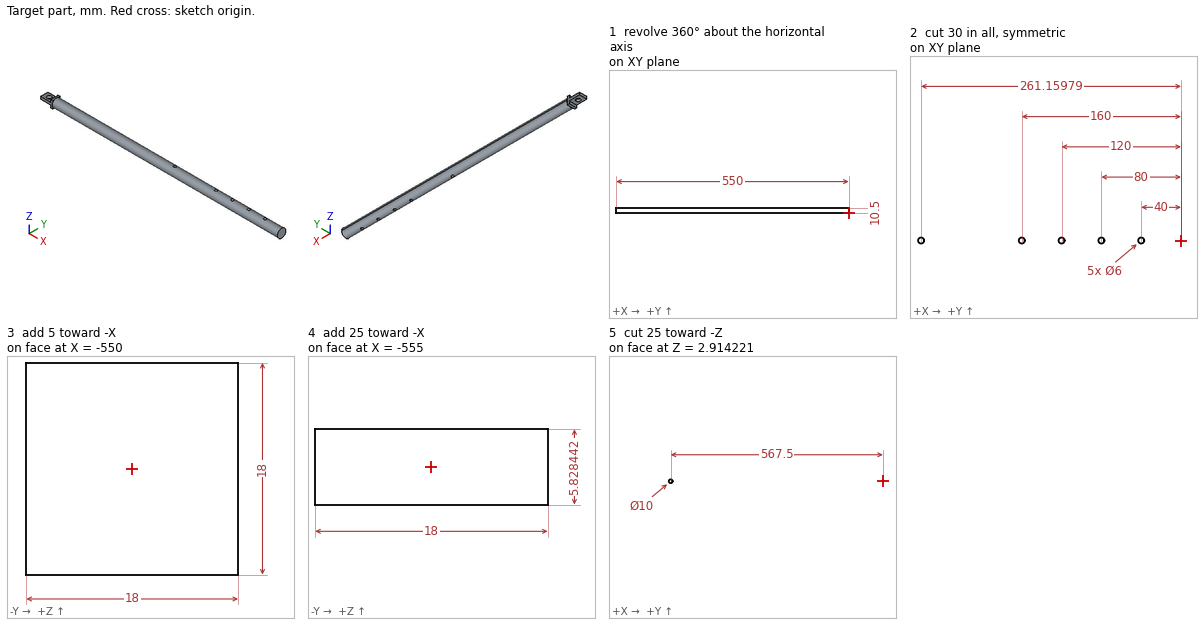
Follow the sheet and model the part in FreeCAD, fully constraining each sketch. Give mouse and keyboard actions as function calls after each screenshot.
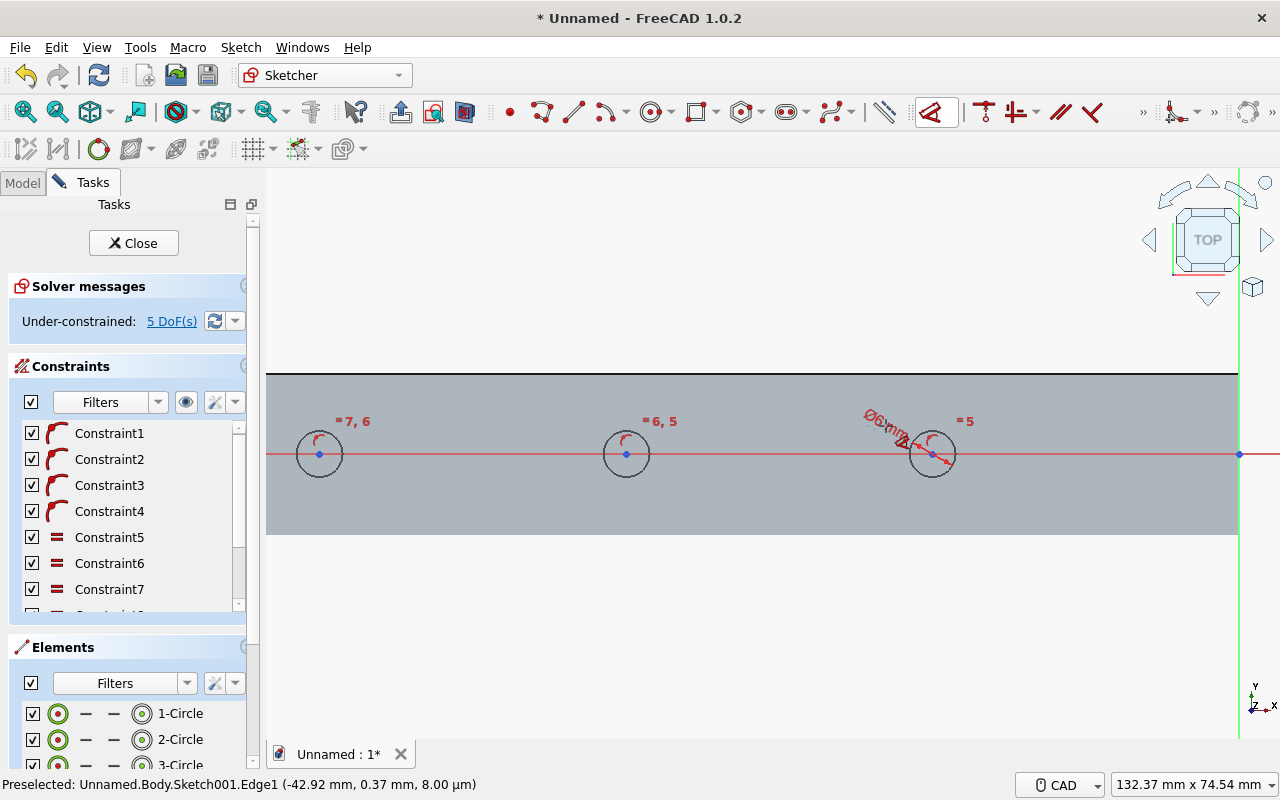
click(933, 454)
click(1024, 488)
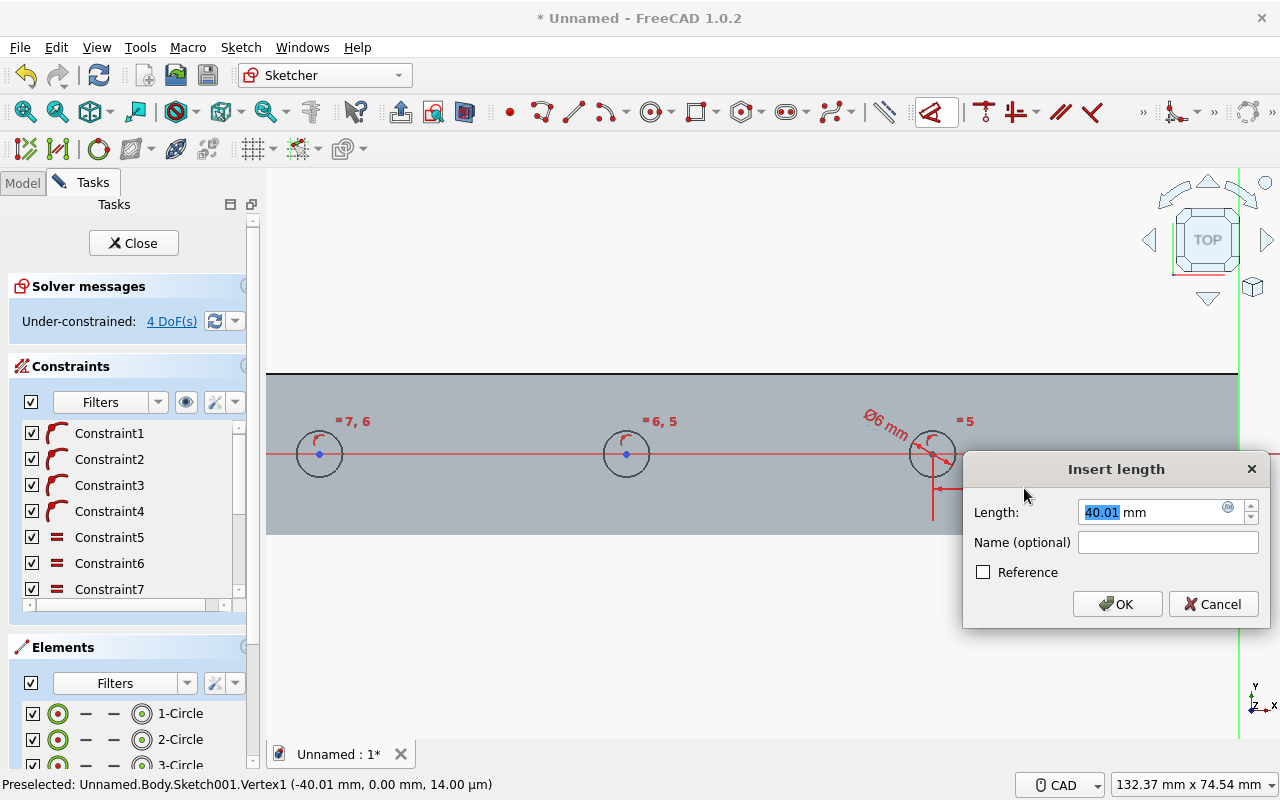
text(40)
key(Return)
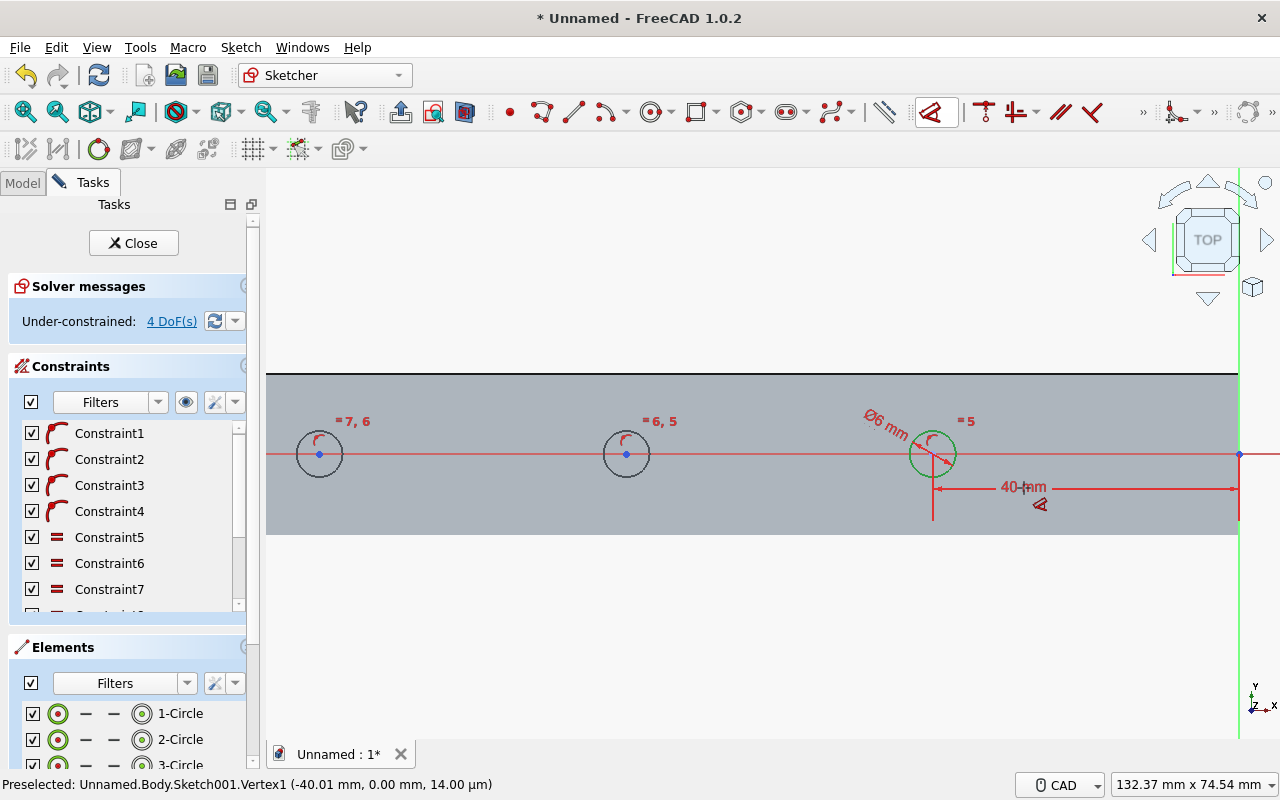
click(627, 454)
click(871, 488)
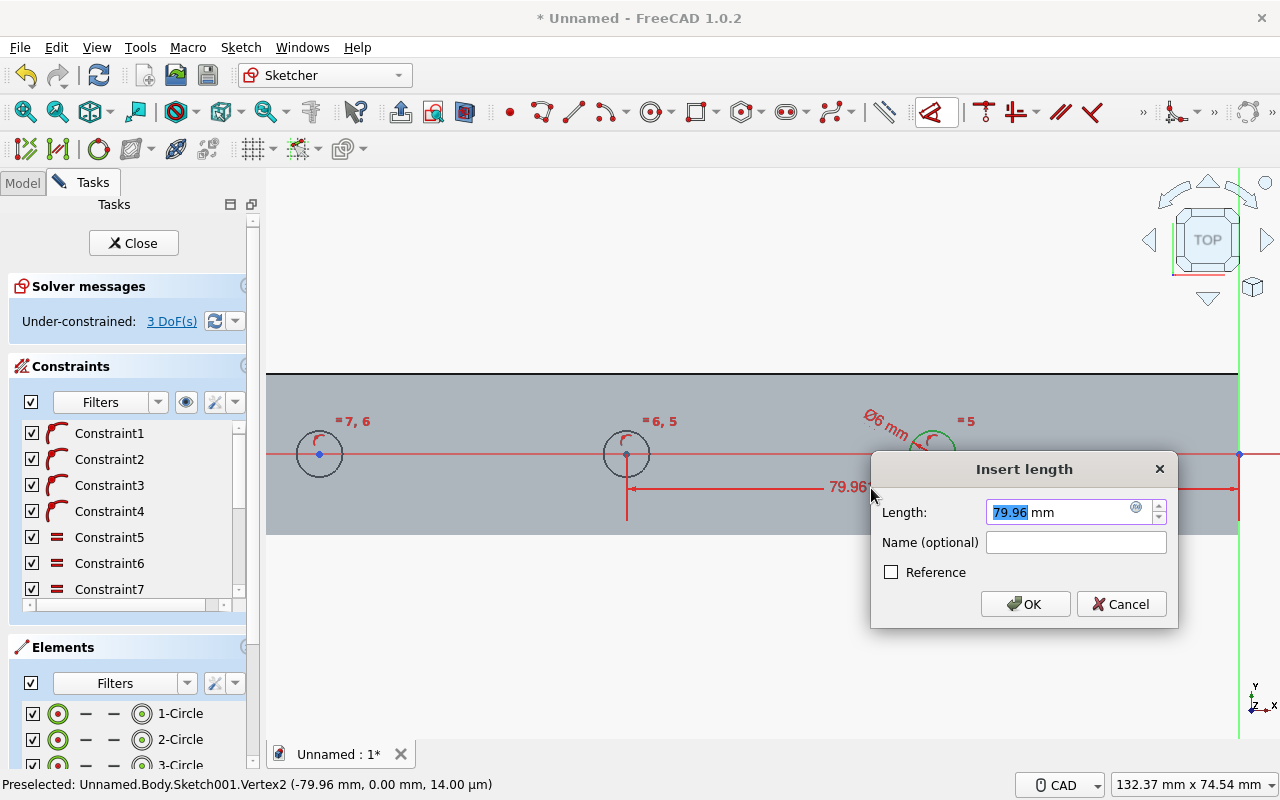
text(80)
key(Return)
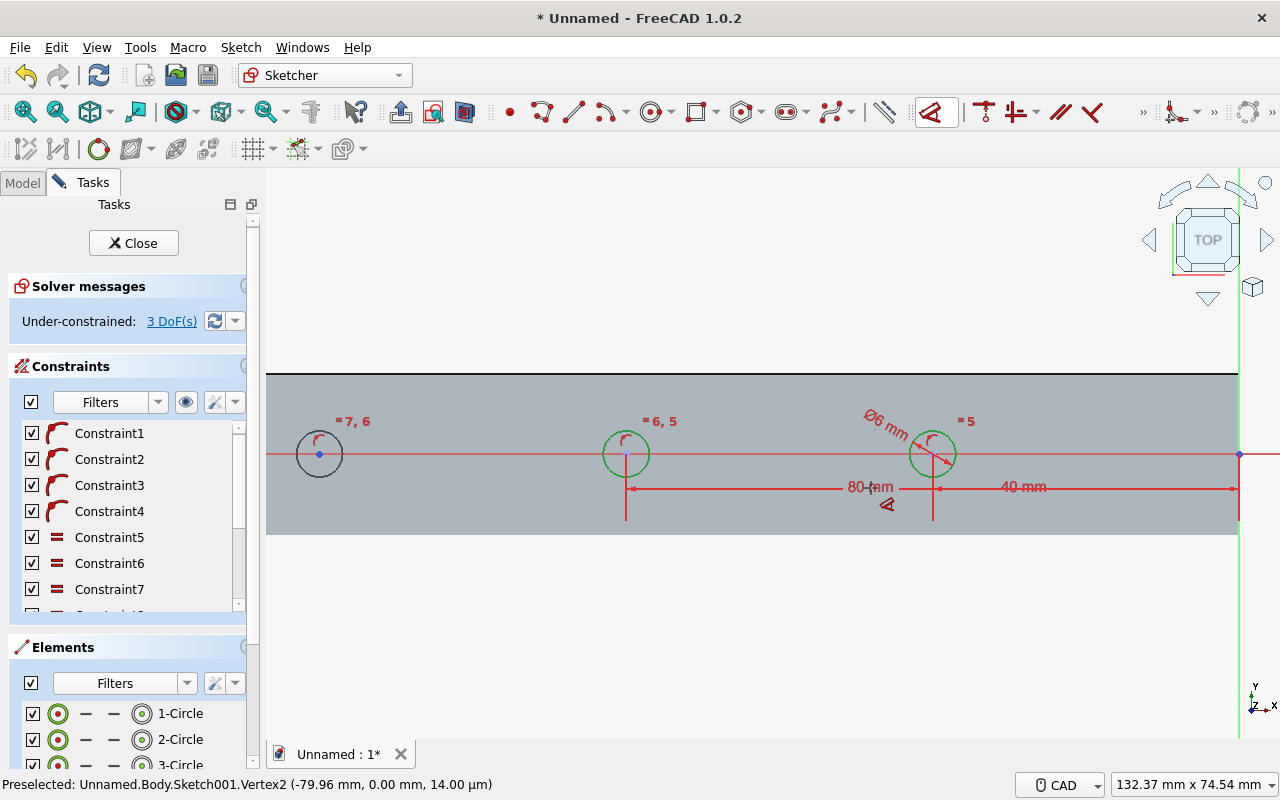
click(320, 454)
click(717, 488)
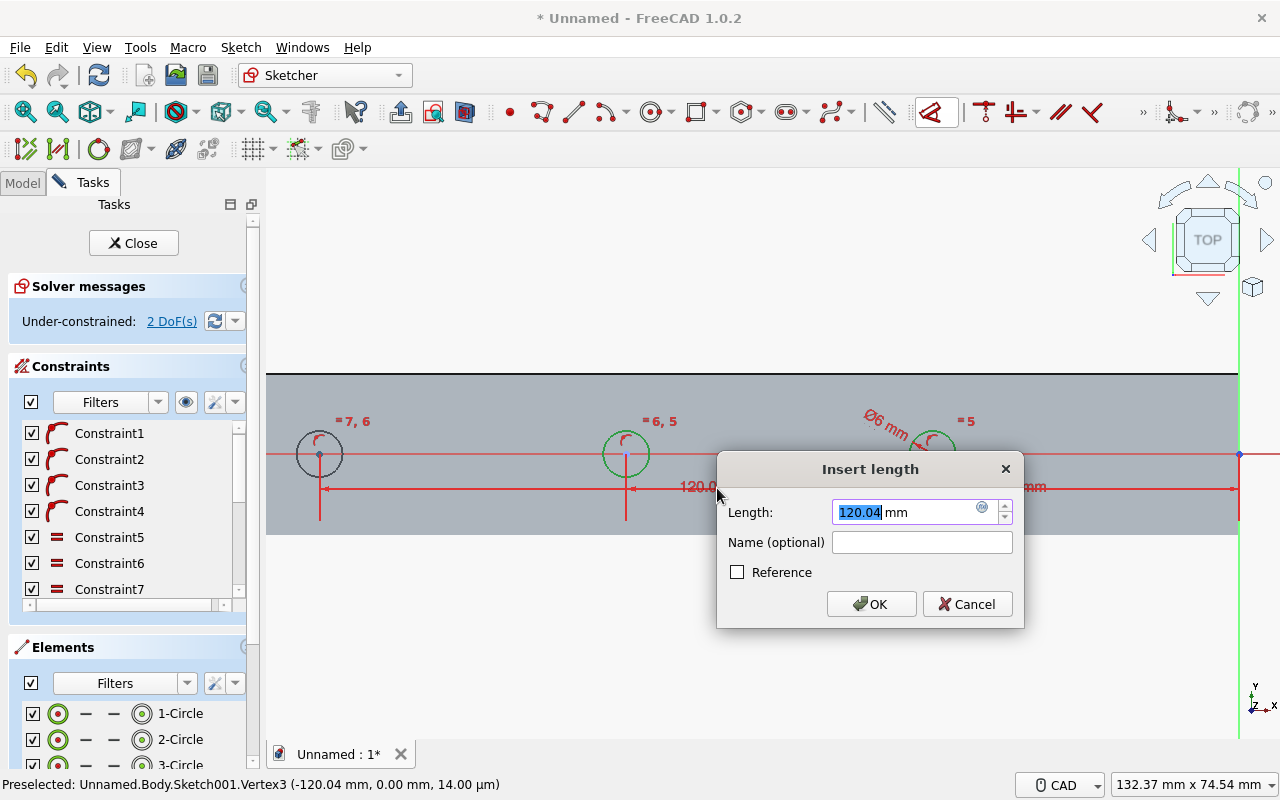
text(120)
key(Return)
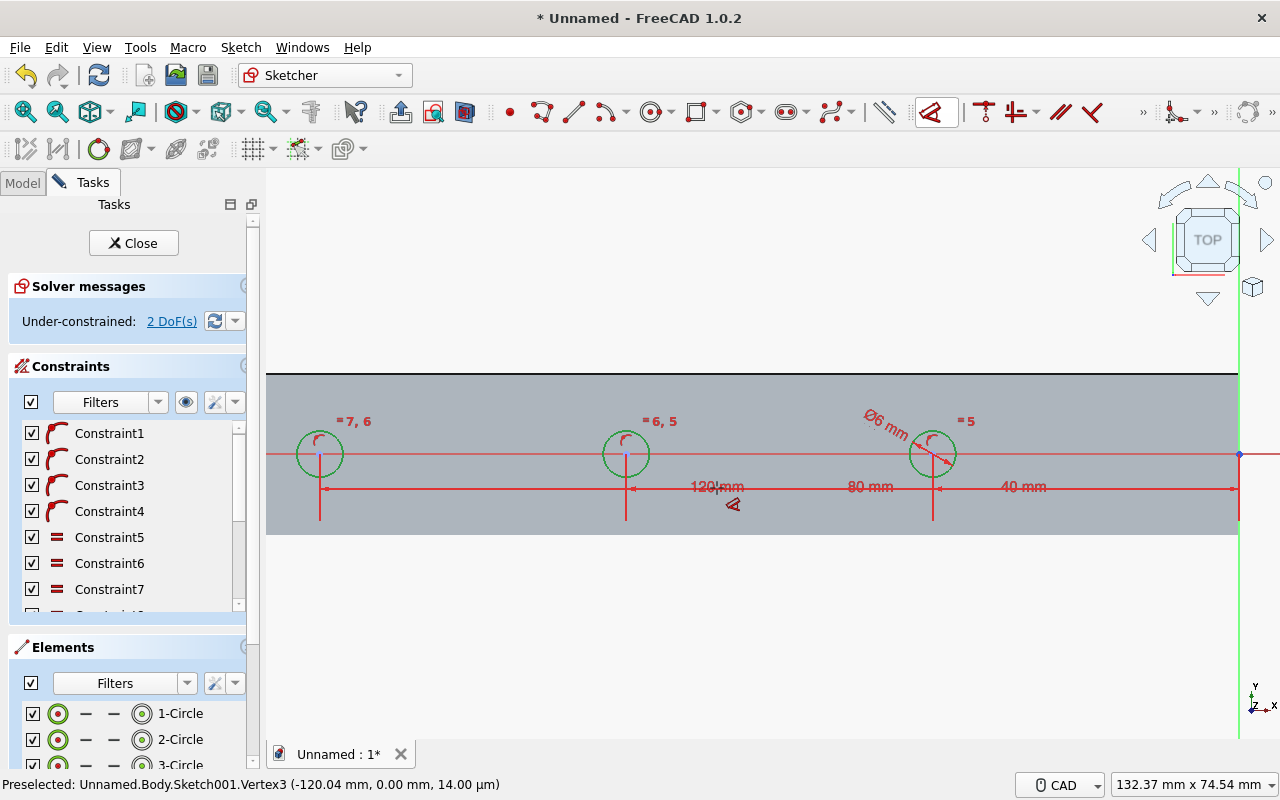
scroll(910, 453, down, 6)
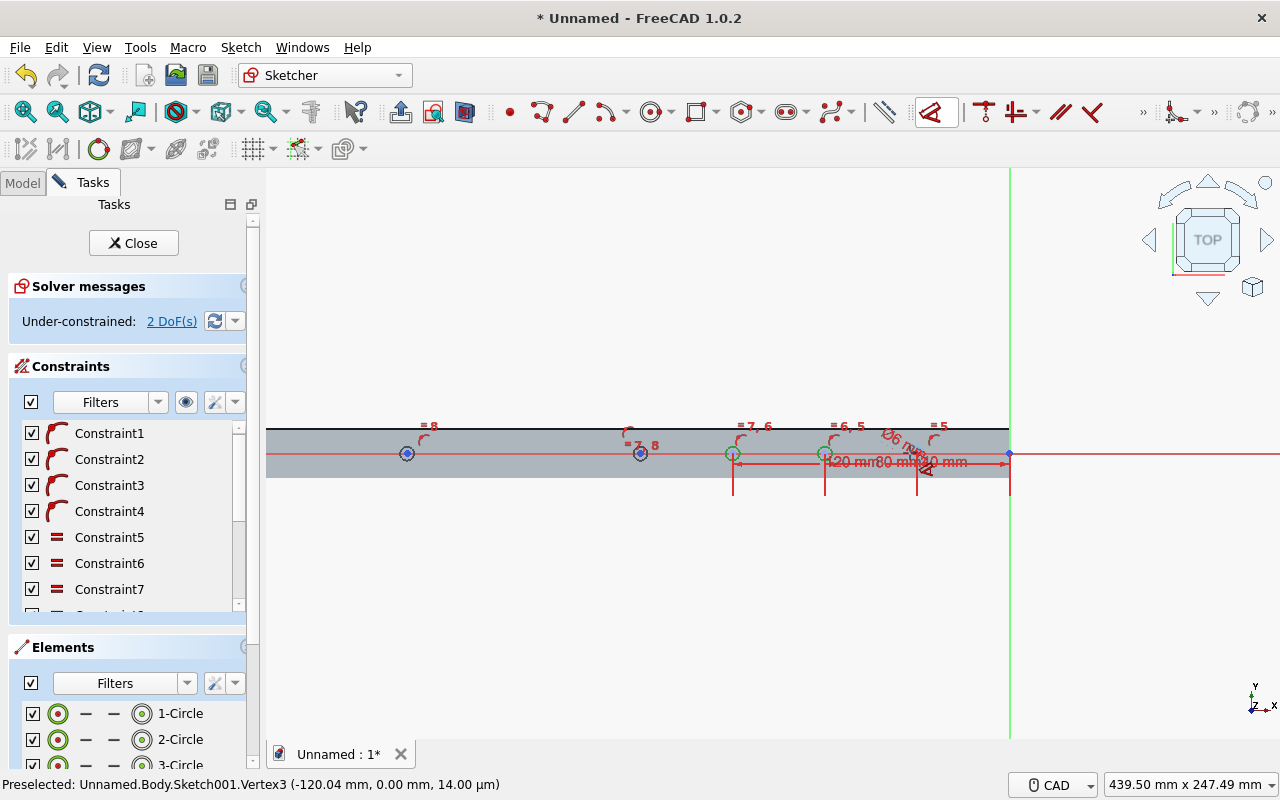
click(641, 454)
click(825, 488)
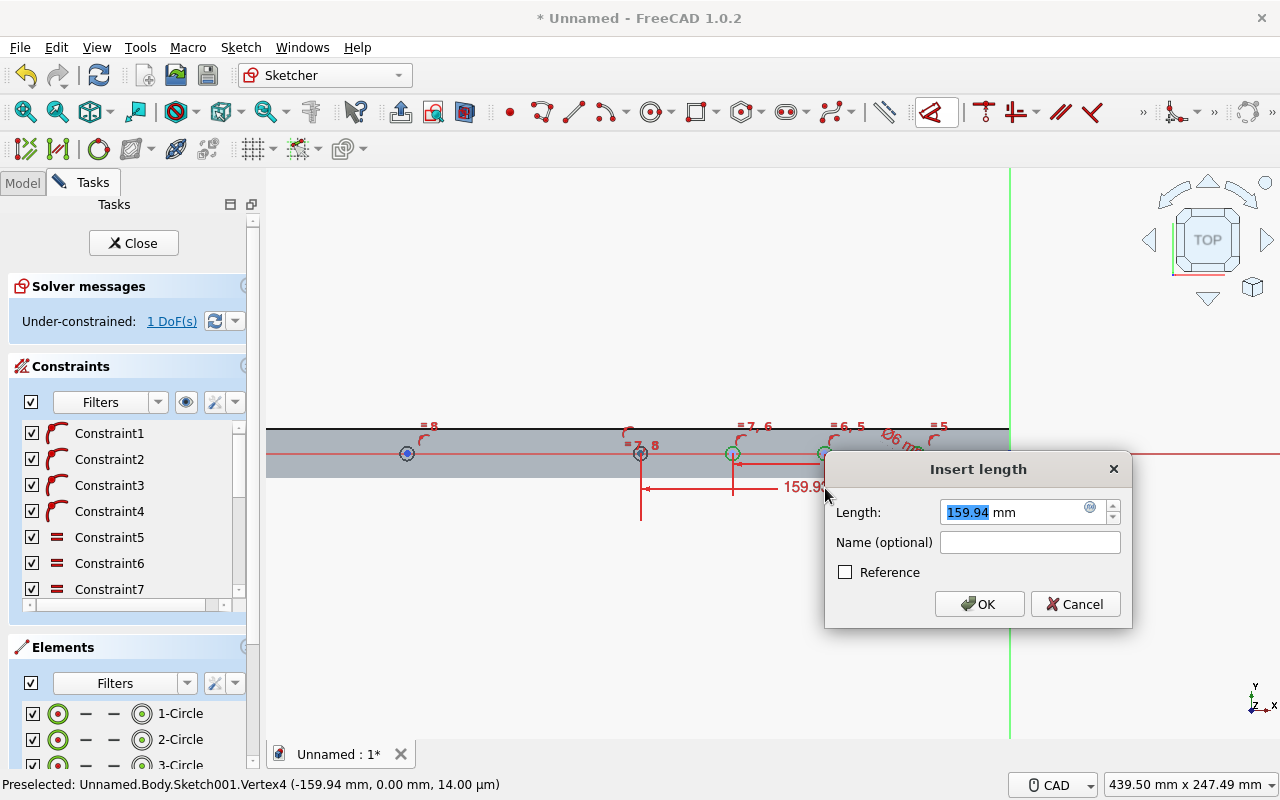
text(160)
key(Return)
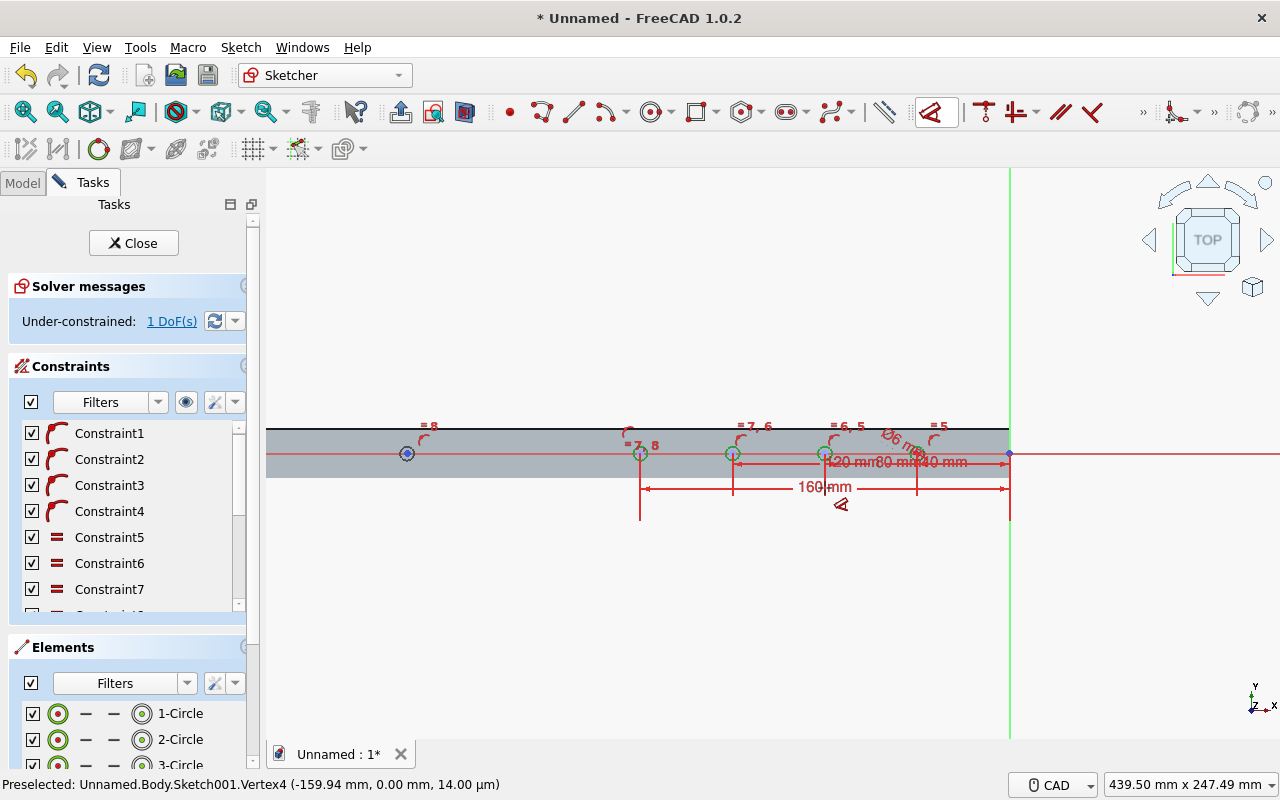
click(407, 454)
click(708, 488)